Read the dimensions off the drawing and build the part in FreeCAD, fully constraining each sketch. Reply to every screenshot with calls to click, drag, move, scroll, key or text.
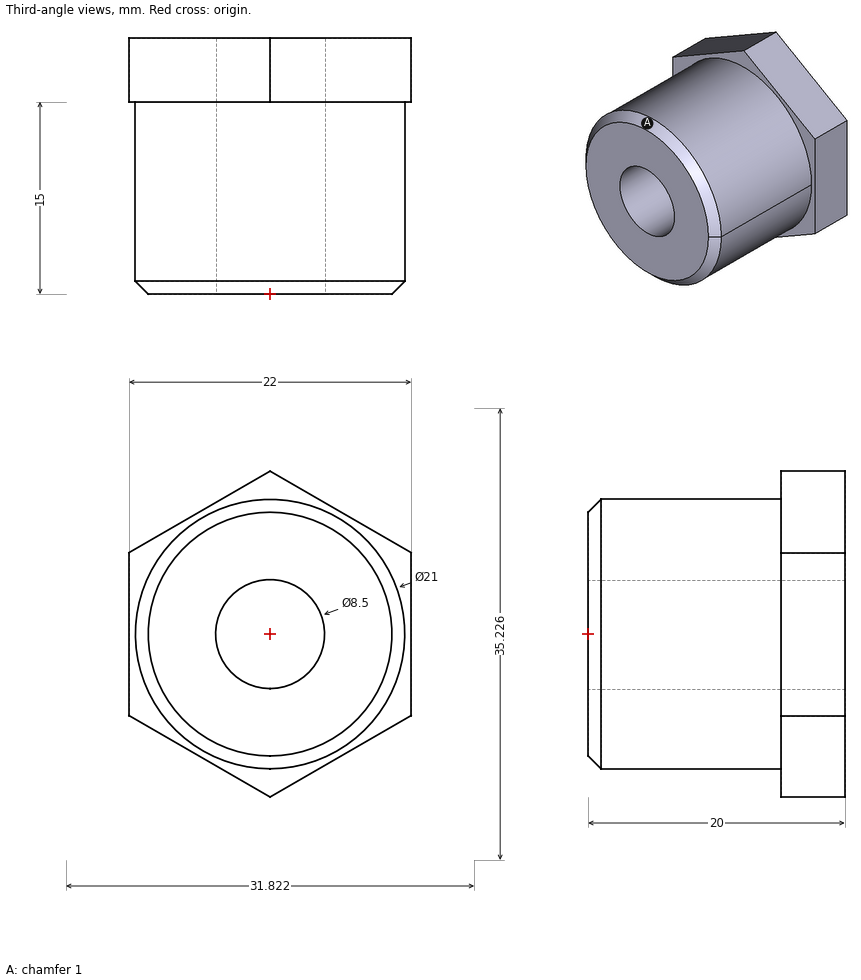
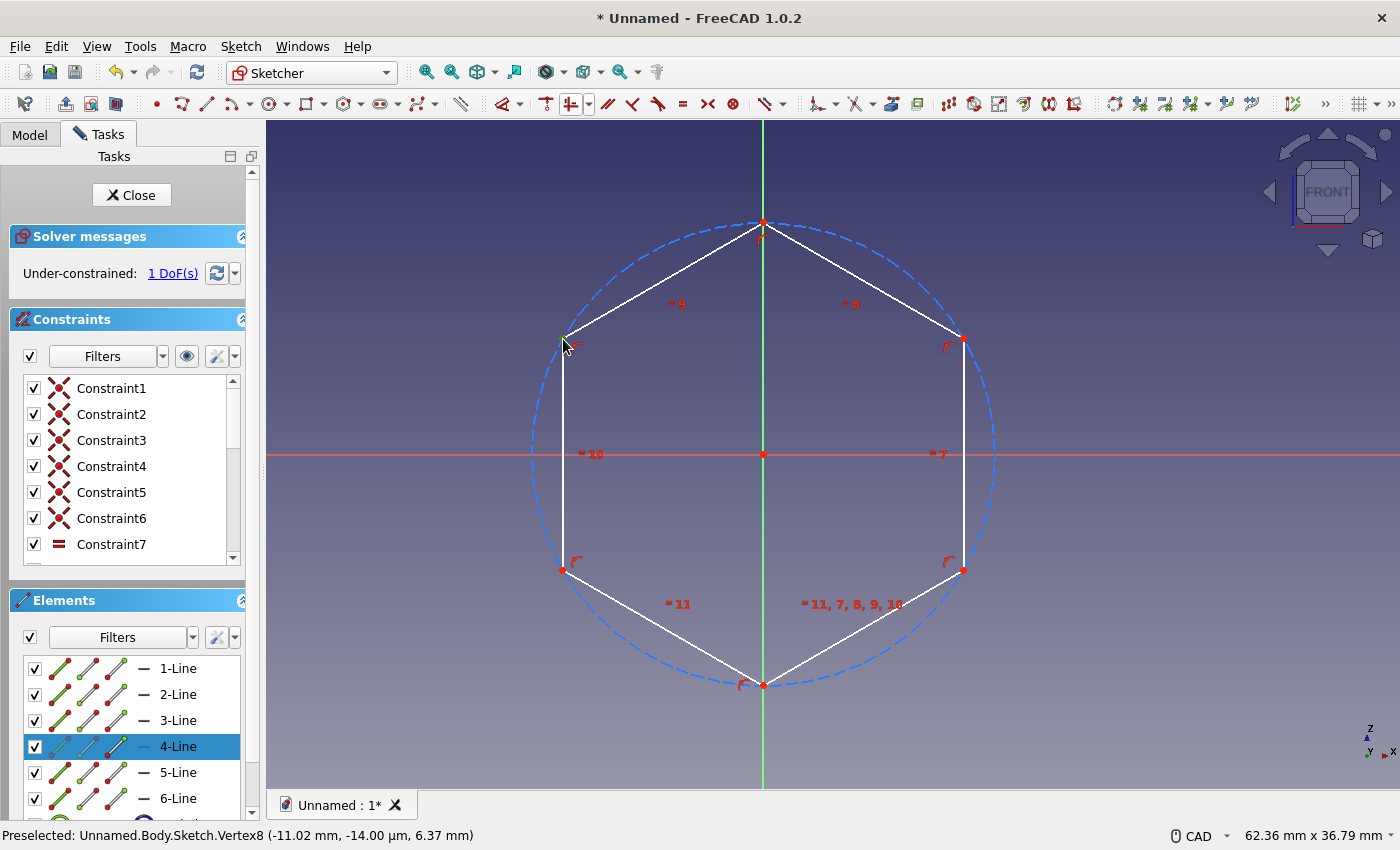
click(964, 570)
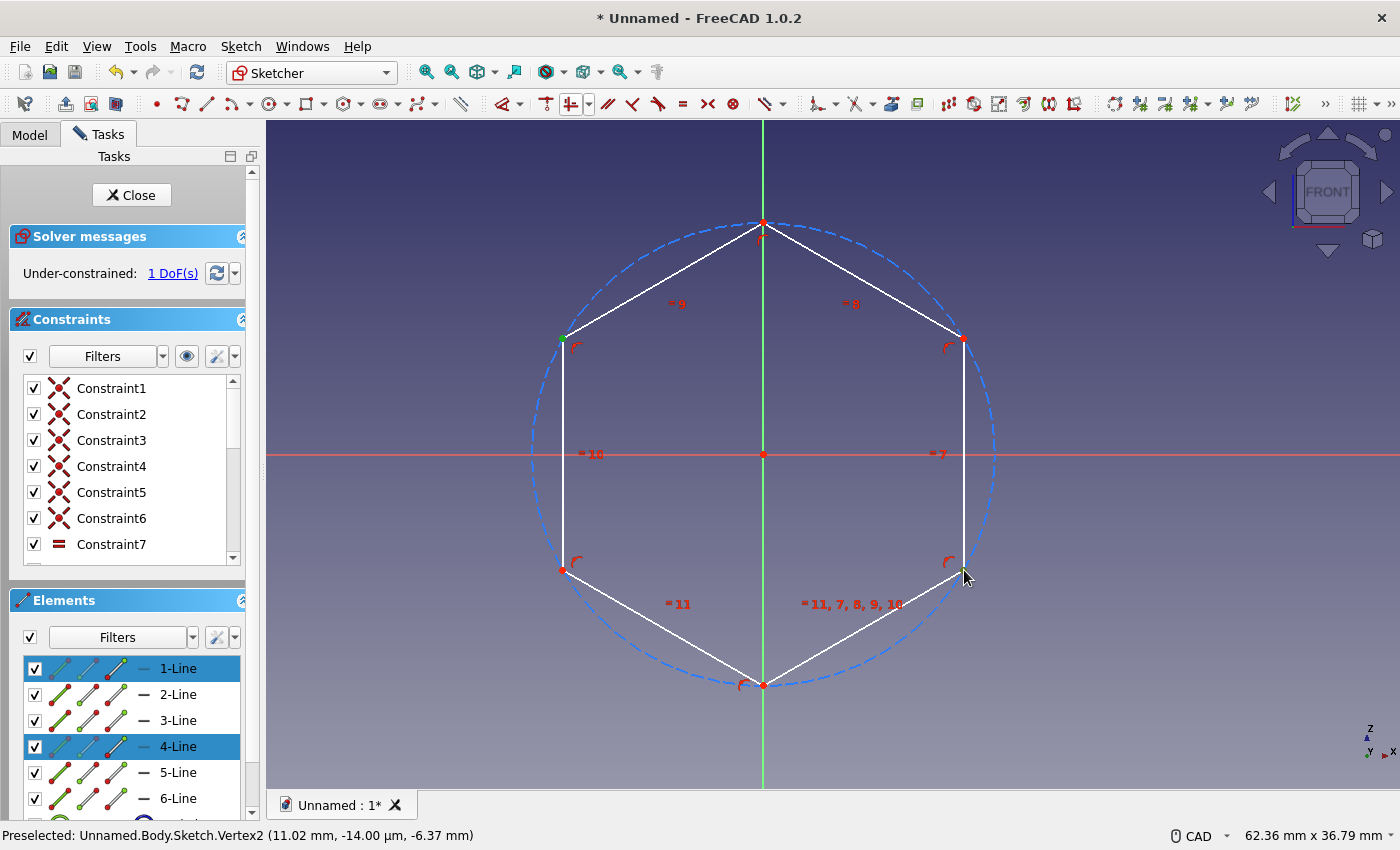
key(l)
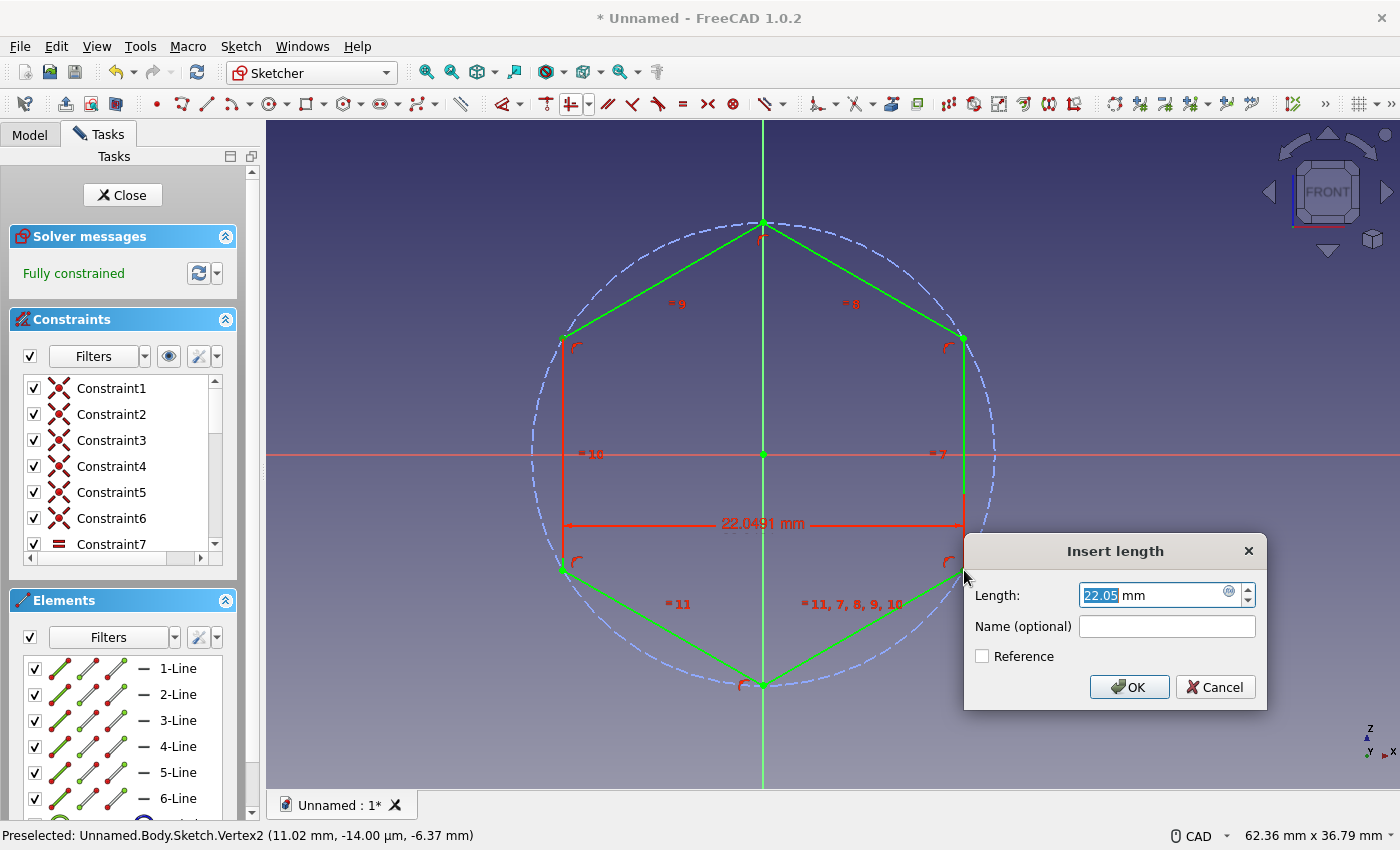
text(22)
key(Return)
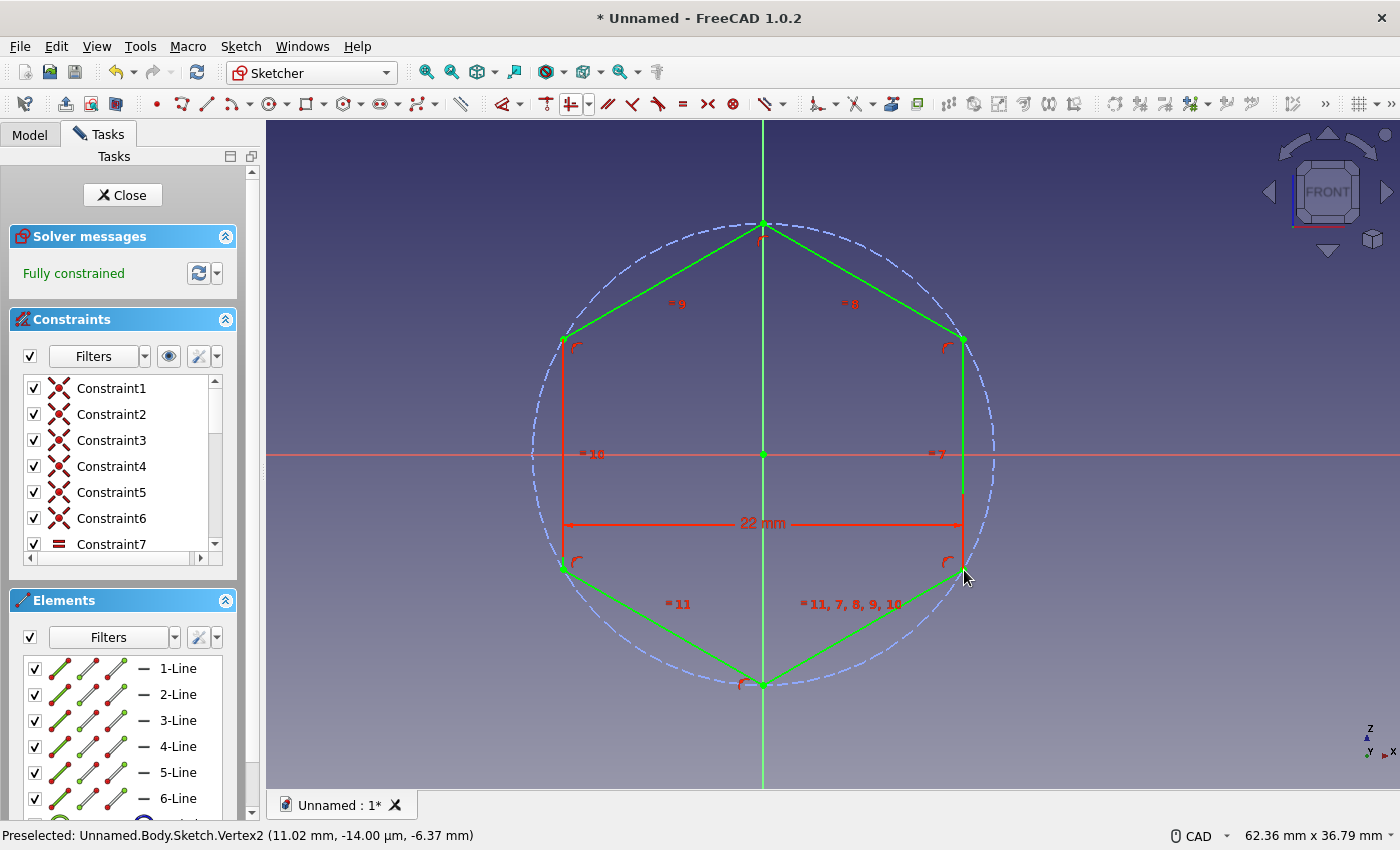
click(123, 195)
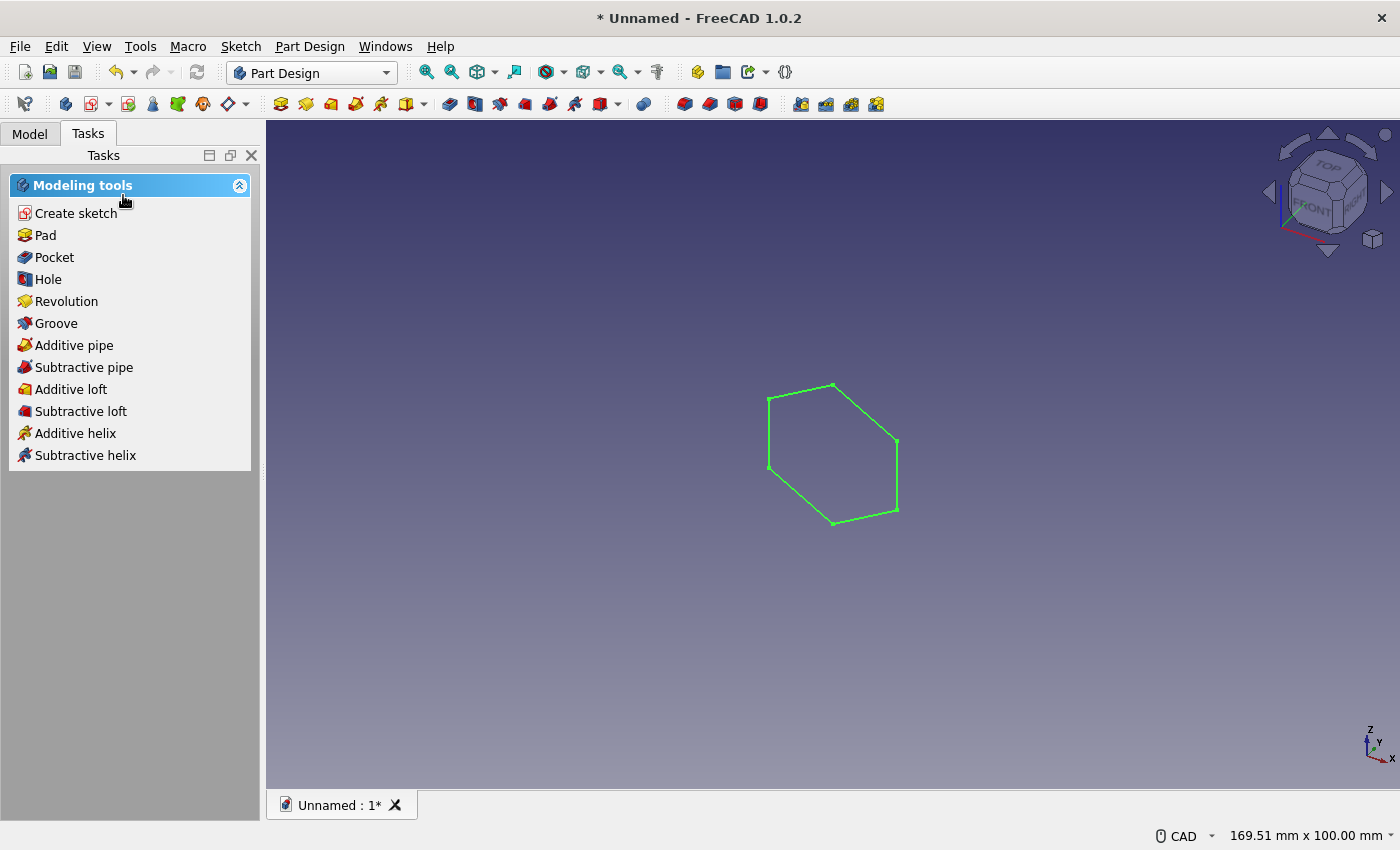
click(281, 104)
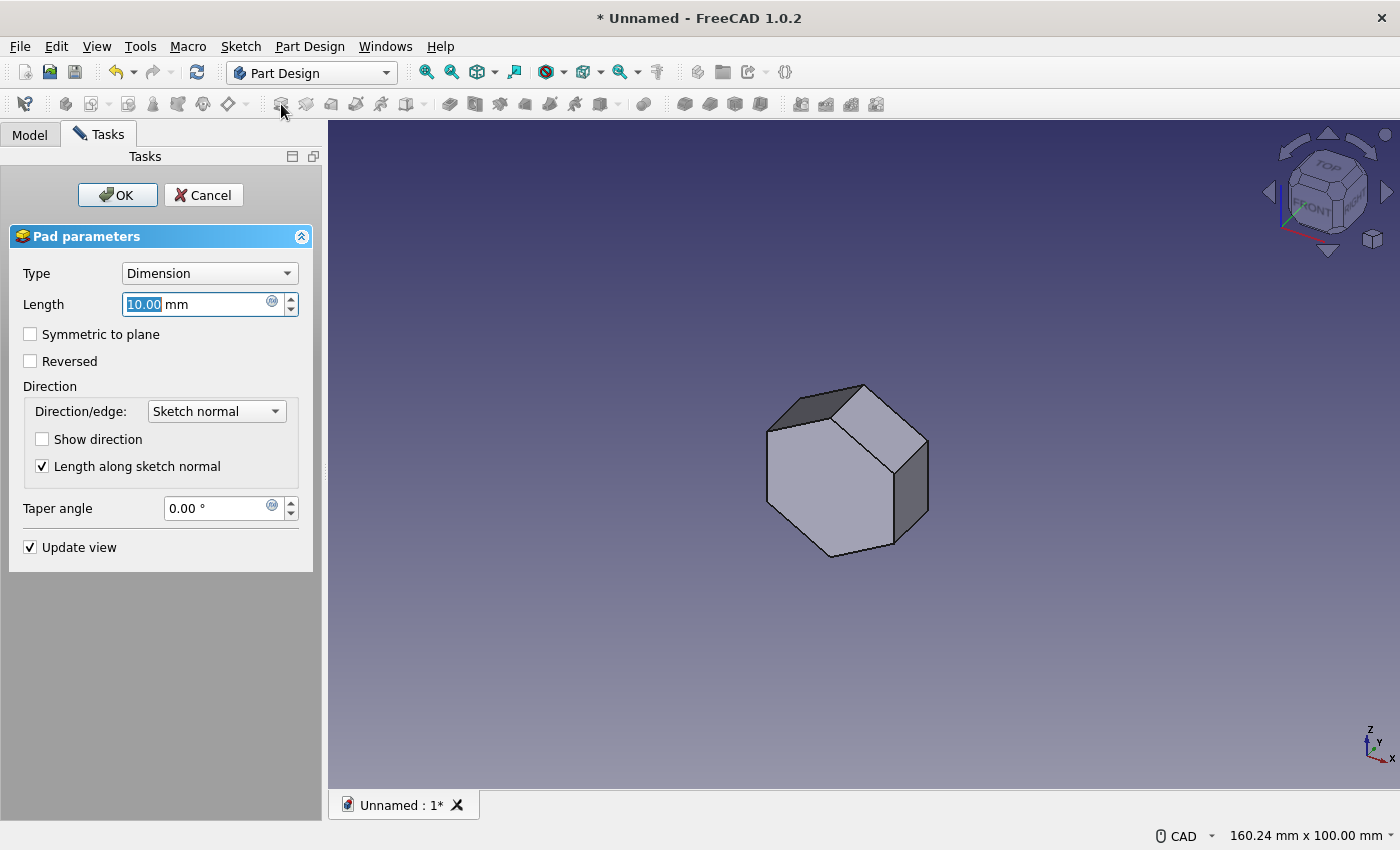
text(20)
key(Tab)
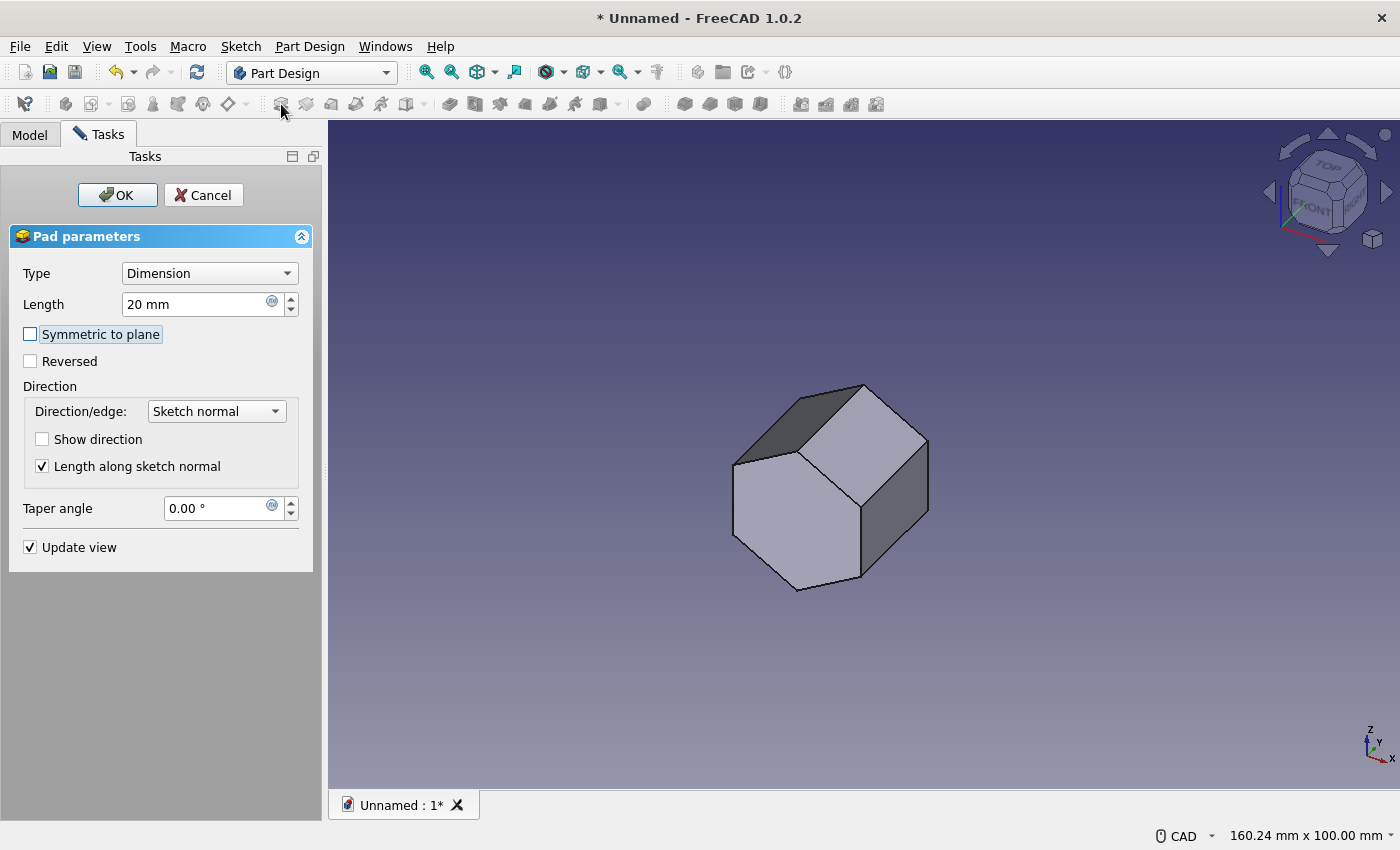
click(31, 361)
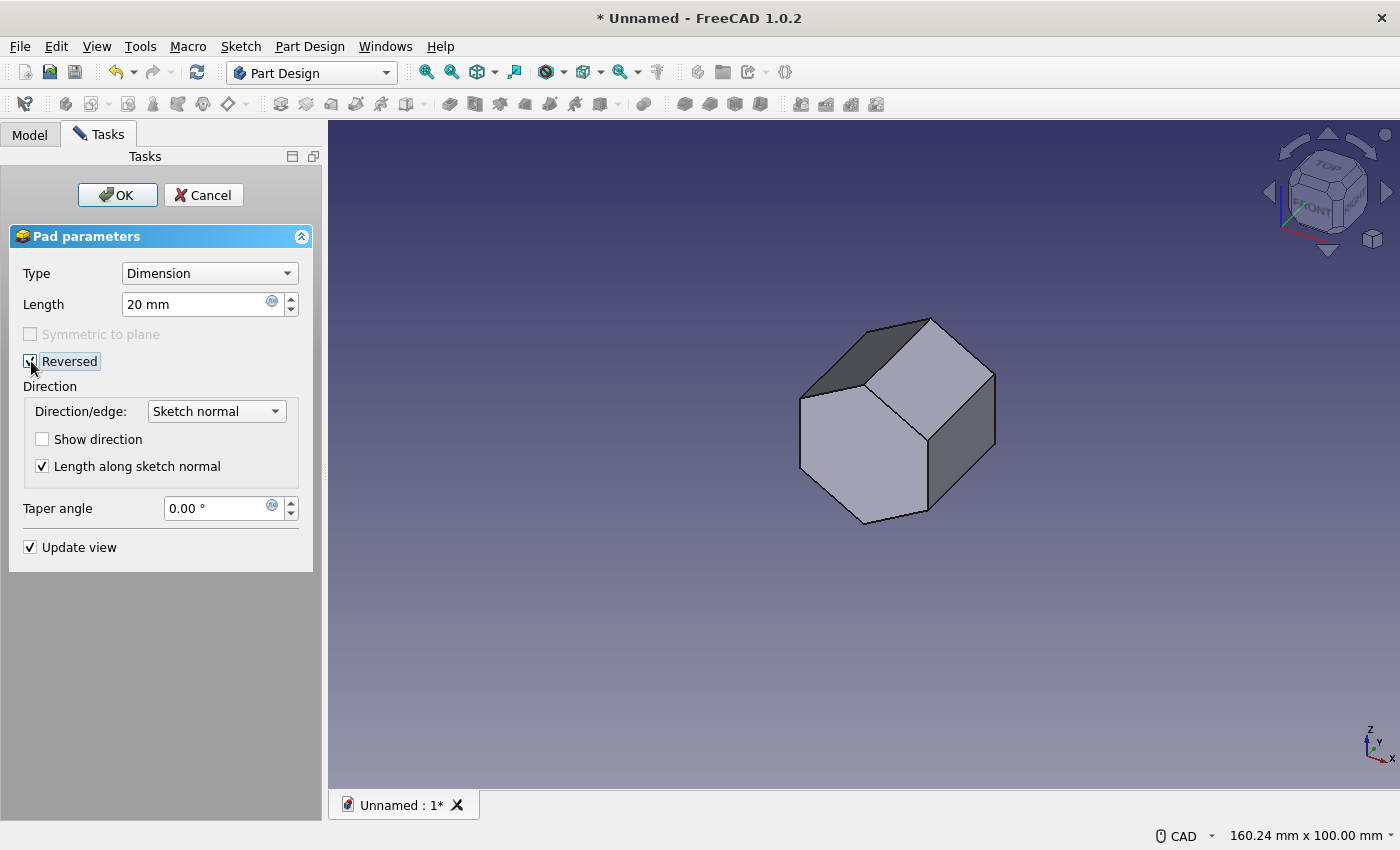
click(118, 195)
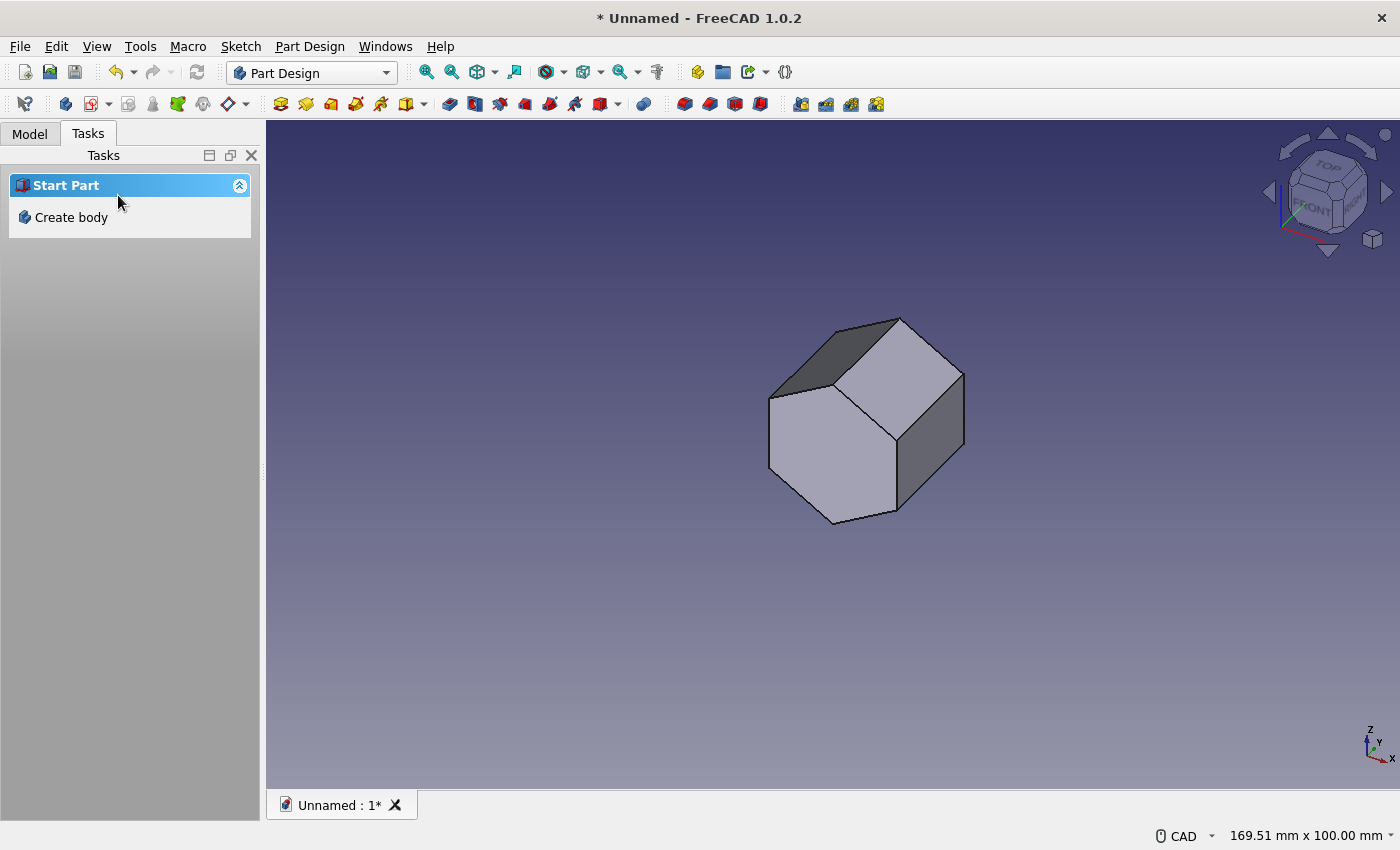
key(v)
key(f)